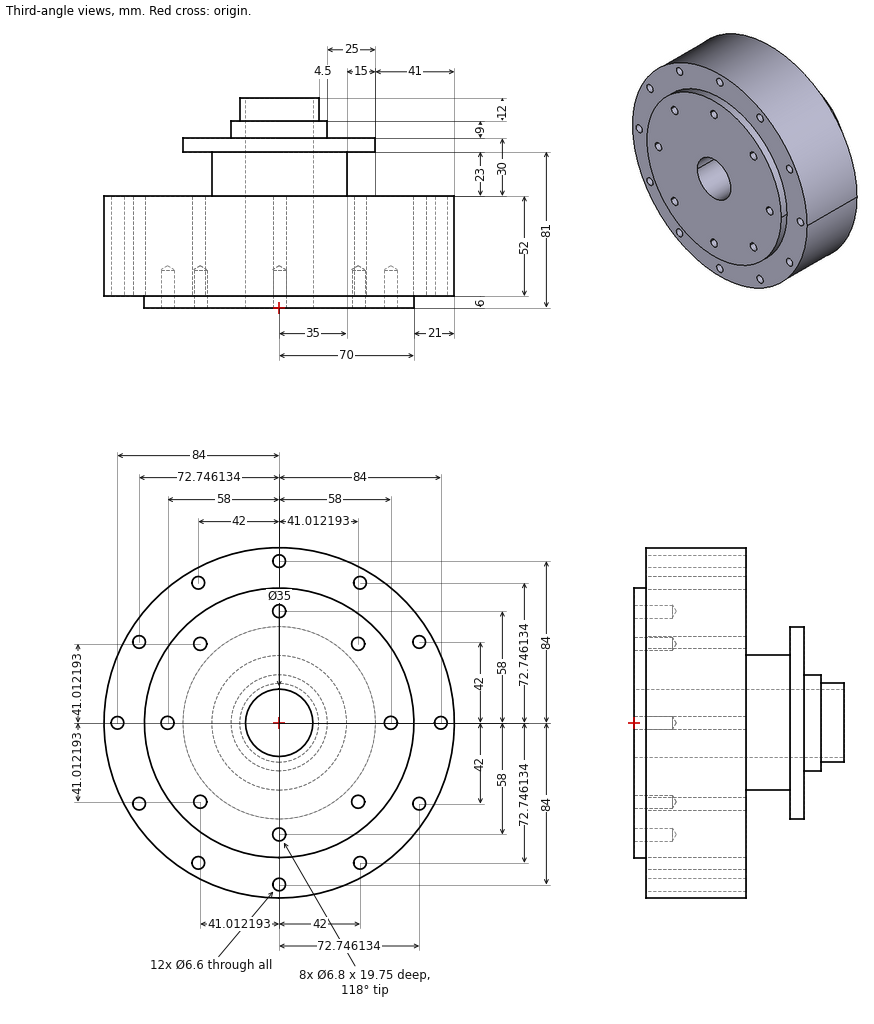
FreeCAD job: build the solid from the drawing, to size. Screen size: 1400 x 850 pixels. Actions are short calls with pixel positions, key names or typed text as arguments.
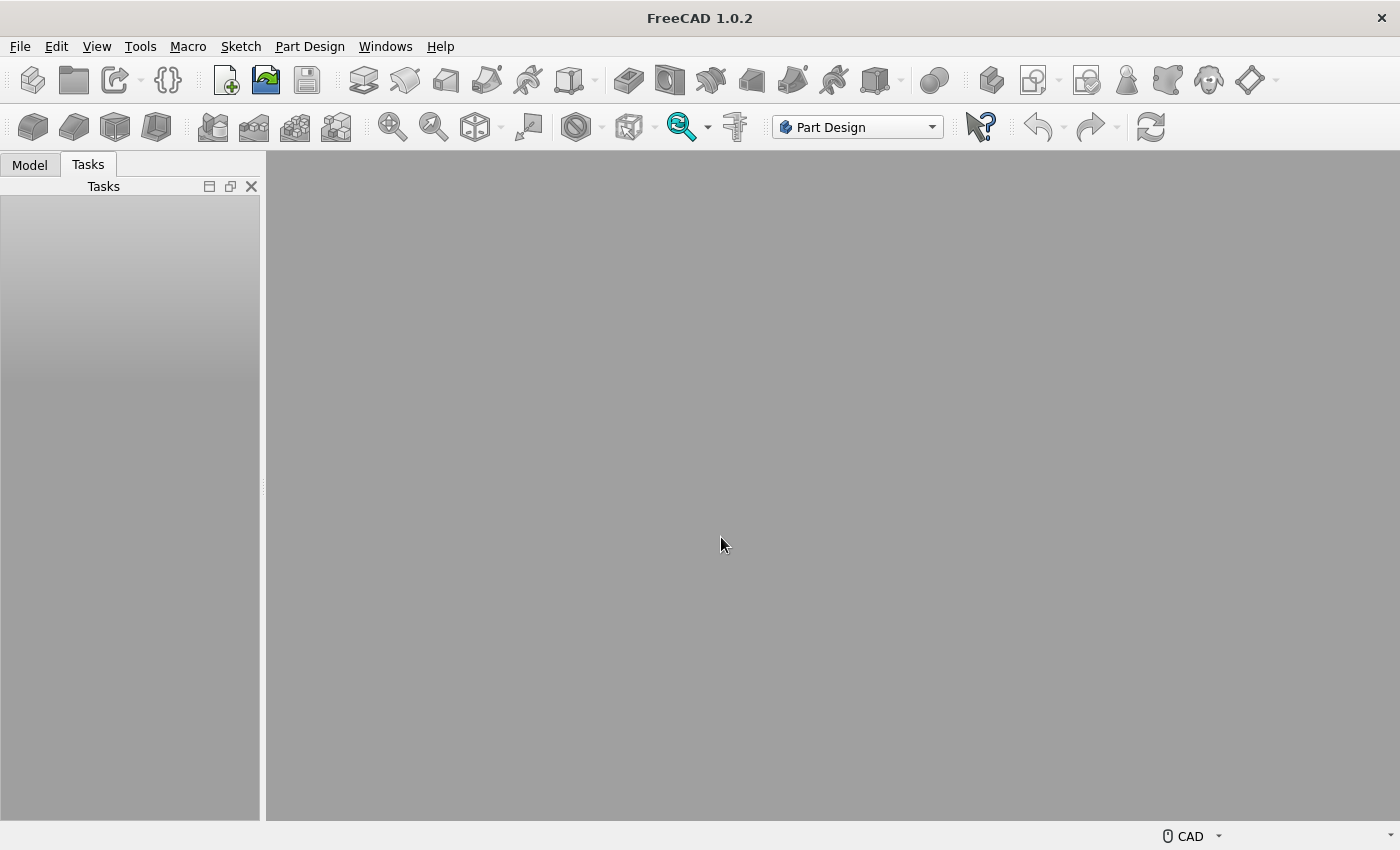
key(ctrl+n)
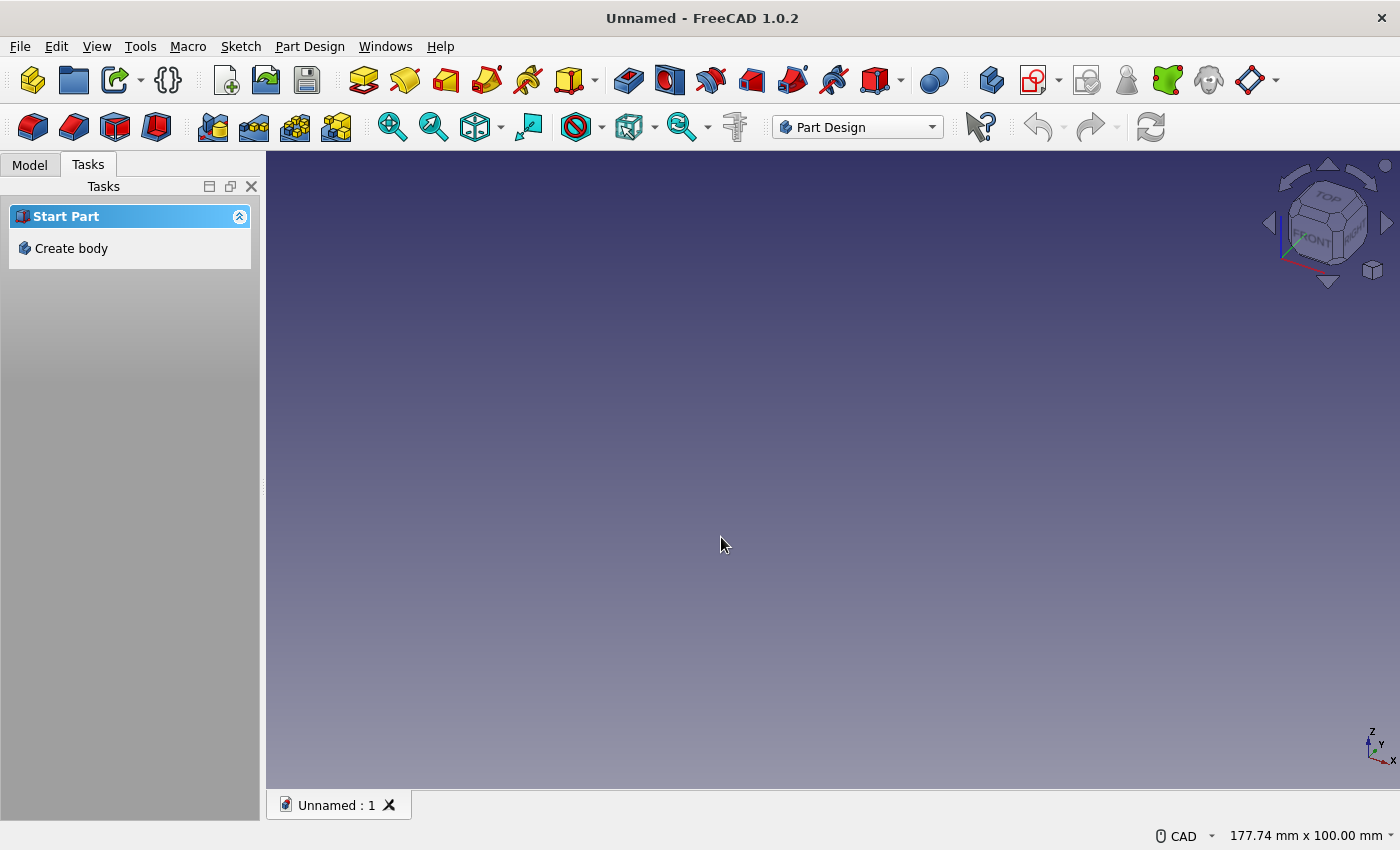
click(1032, 80)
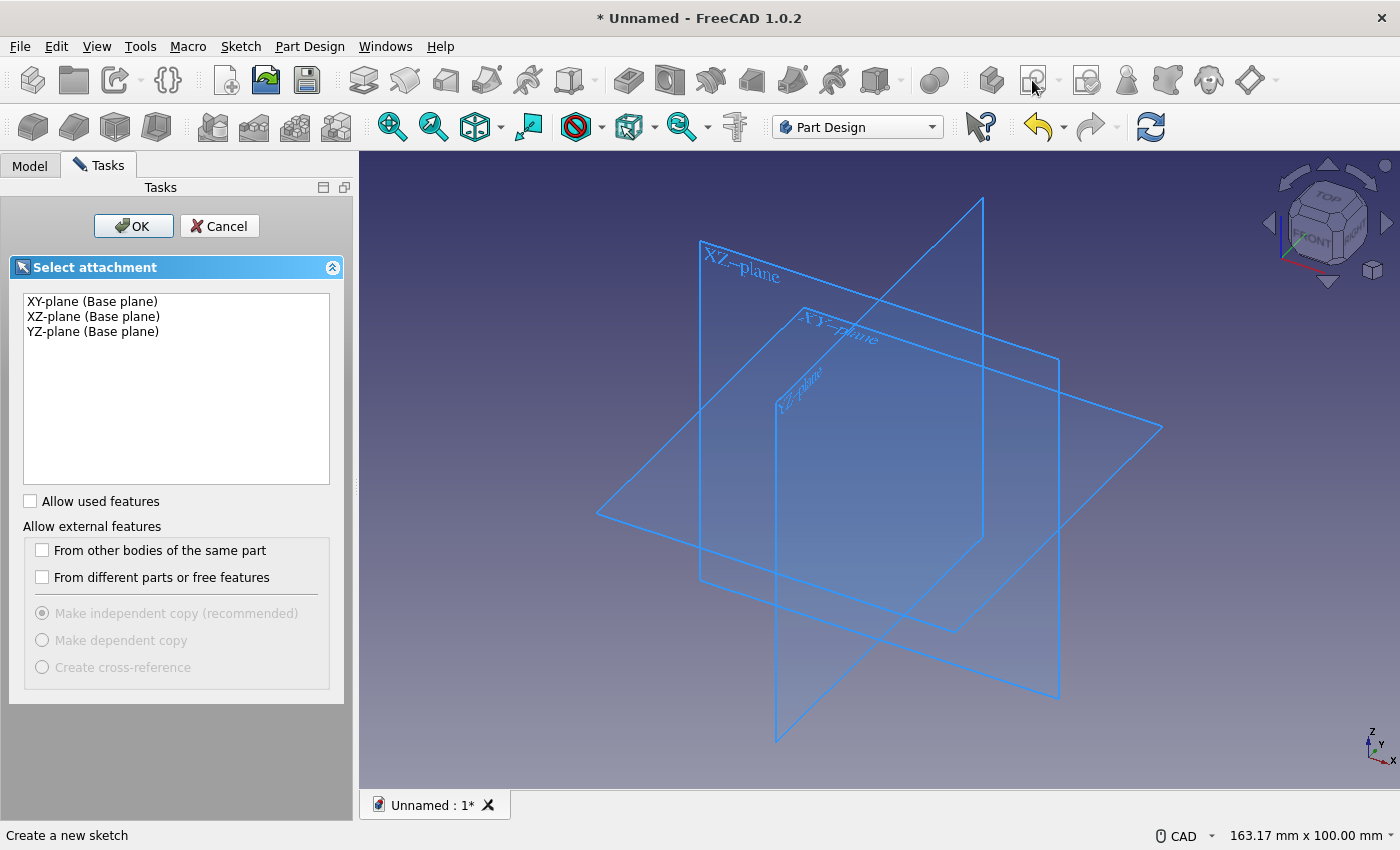
click(84, 302)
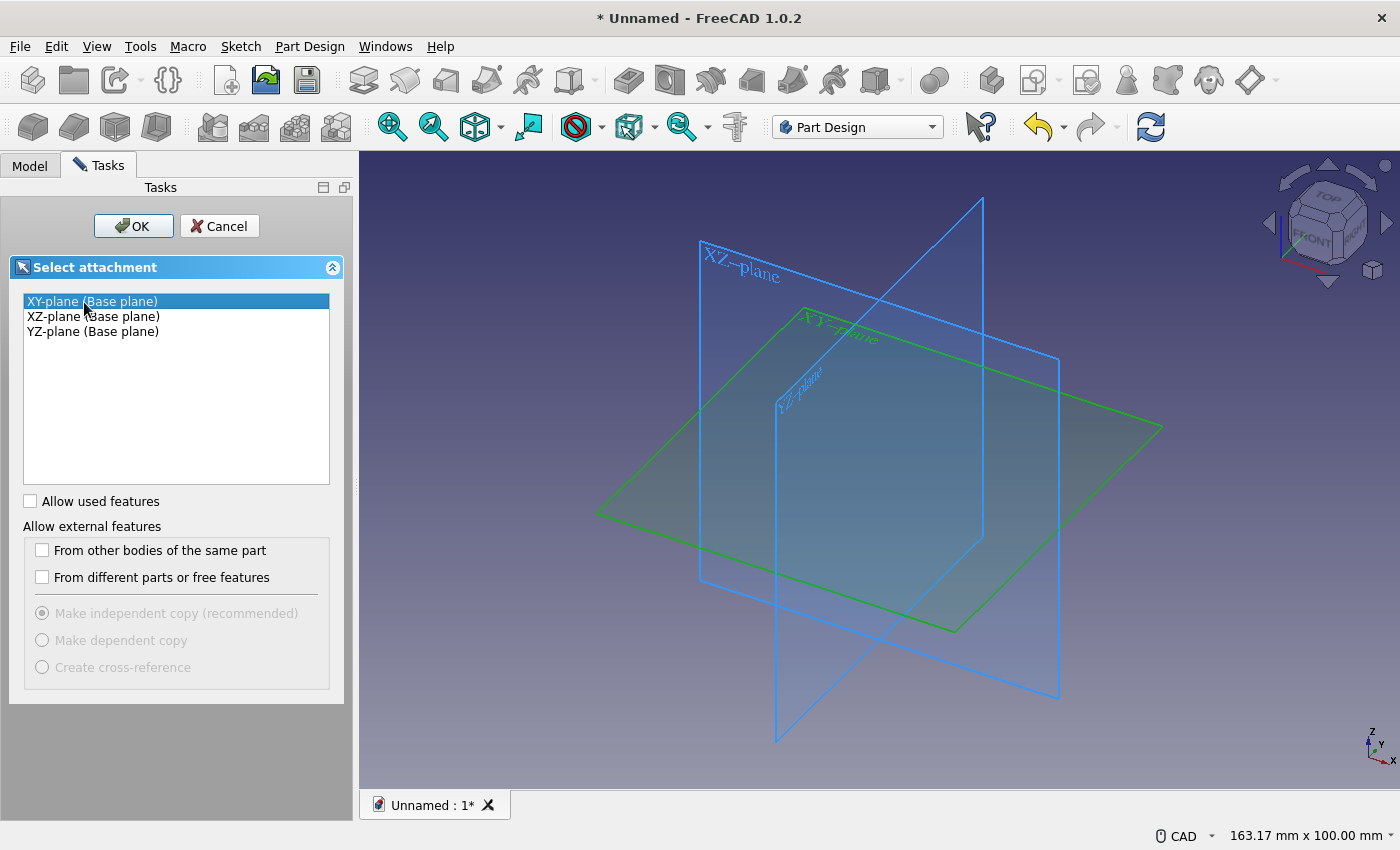
click(134, 226)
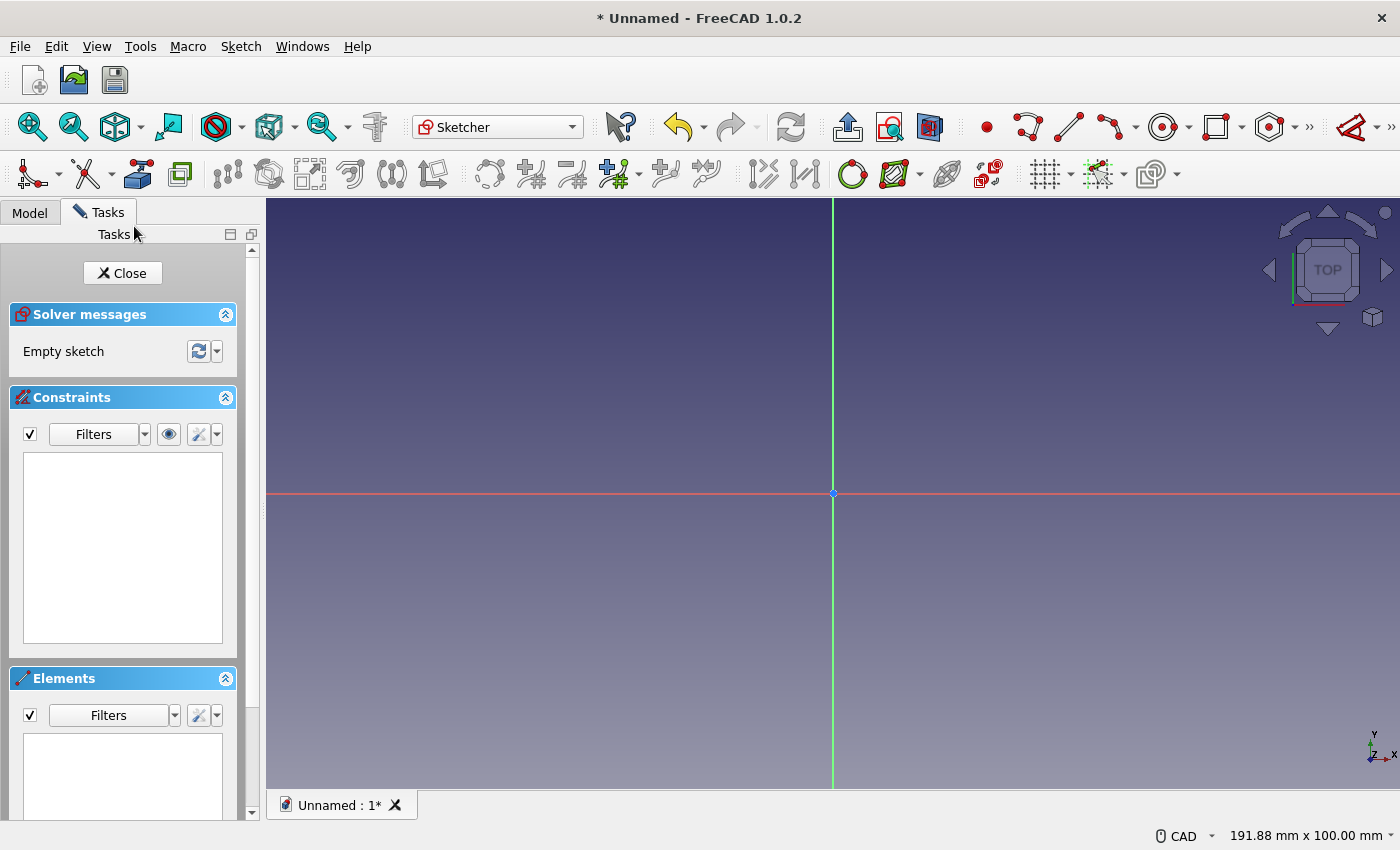
scroll(354, 761, down, 3)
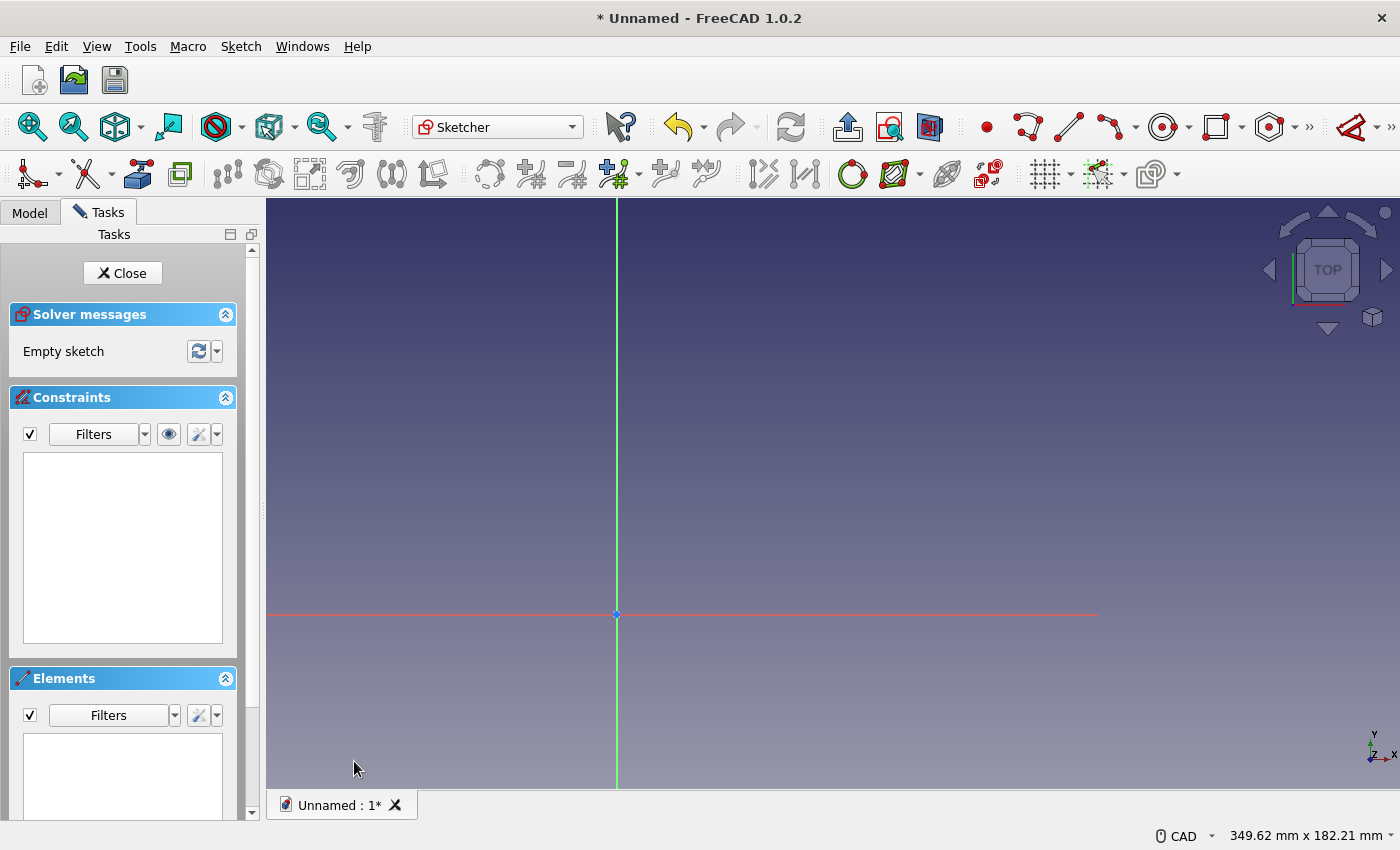
key(g)
key(m)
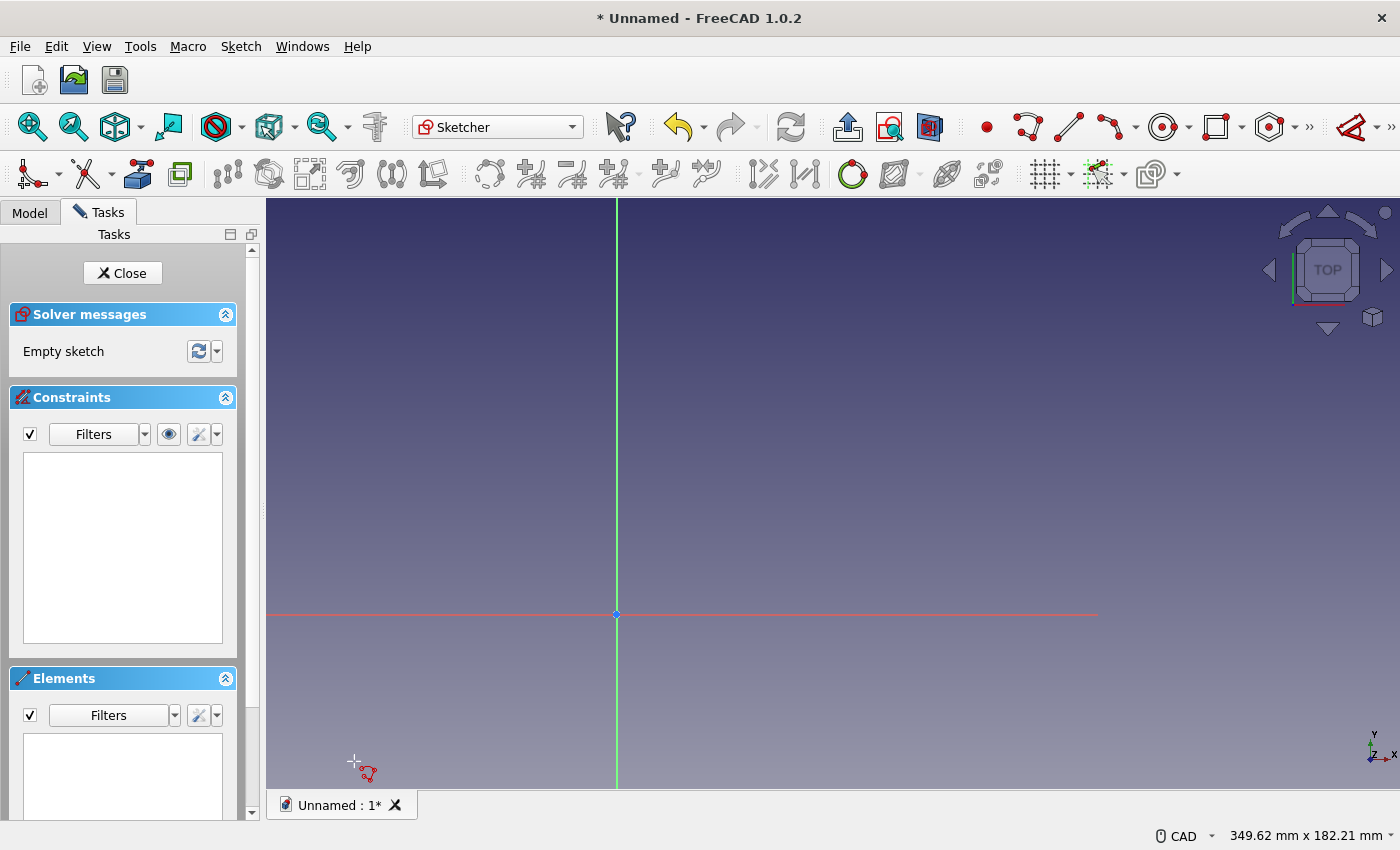
click(617, 615)
click(844, 606)
click(844, 595)
click(912, 595)
click(912, 427)
click(779, 427)
click(779, 329)
click(698, 329)
click(698, 300)
click(683, 300)
click(683, 261)
click(626, 261)
click(617, 615)
key(Escape)
key(Escape)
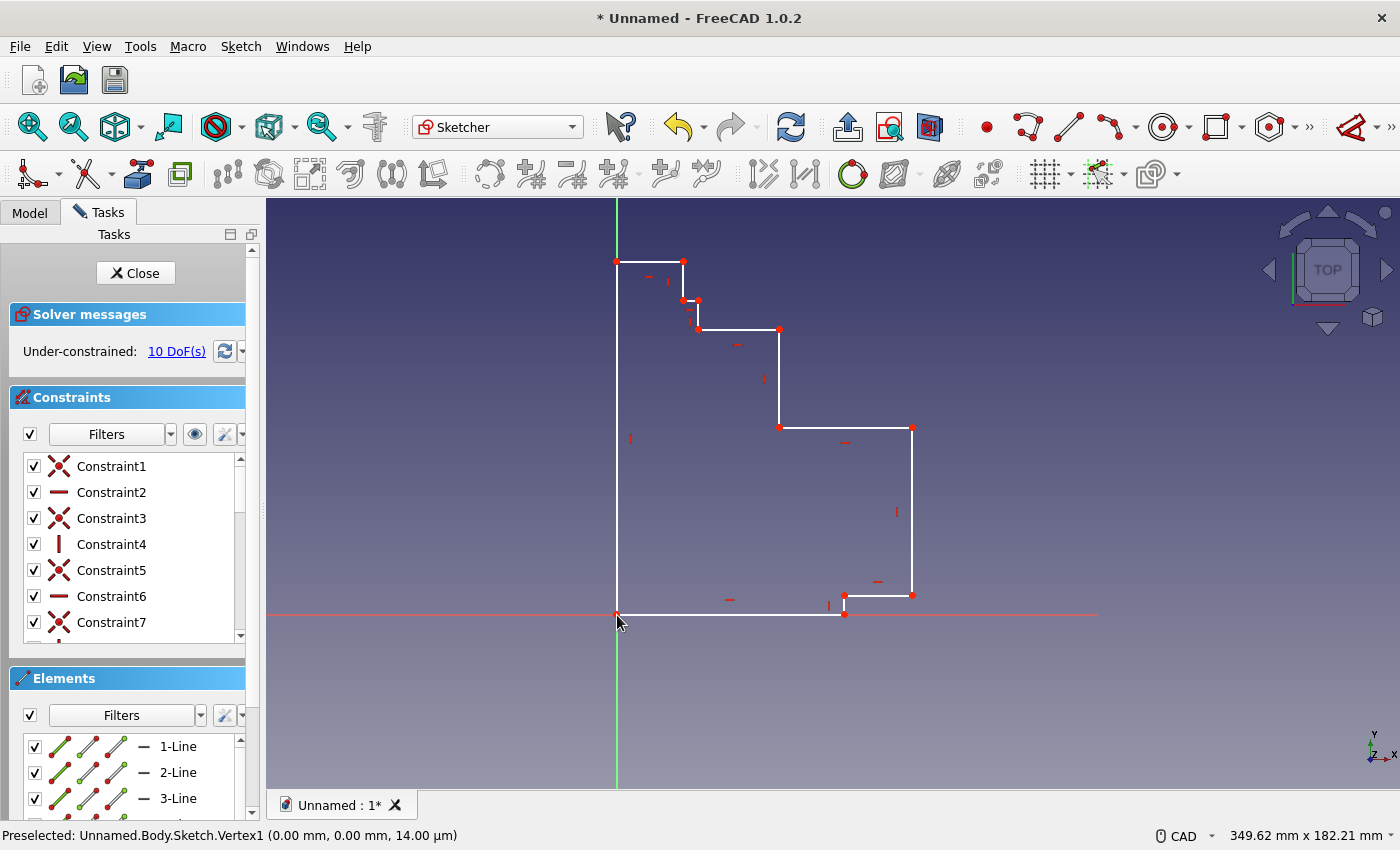
key(d)